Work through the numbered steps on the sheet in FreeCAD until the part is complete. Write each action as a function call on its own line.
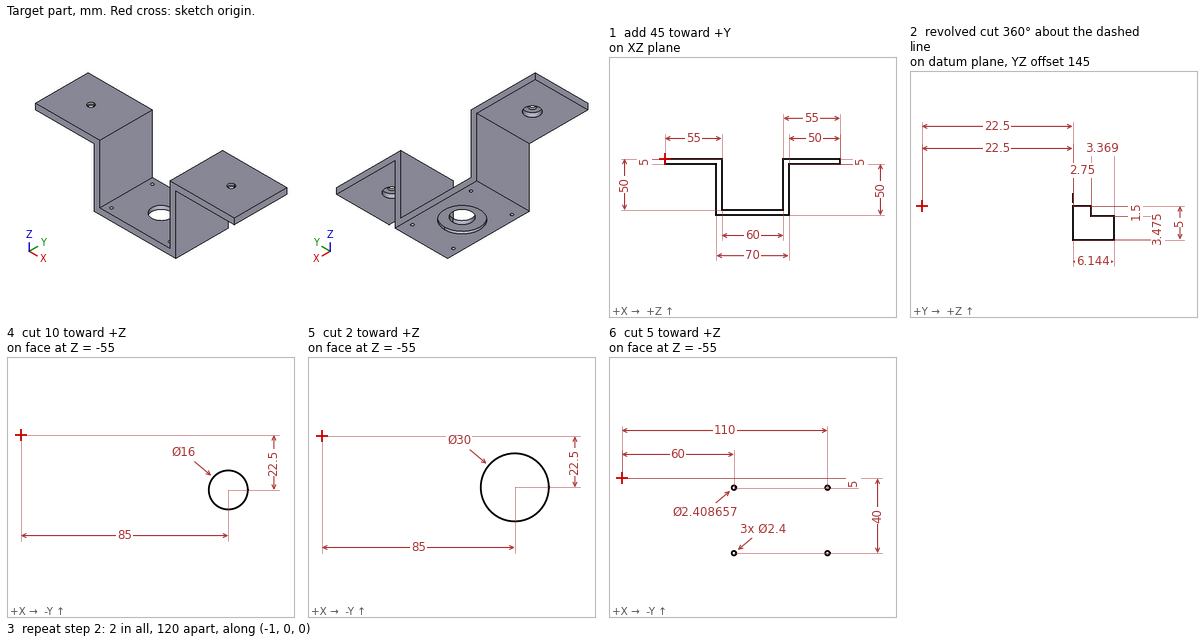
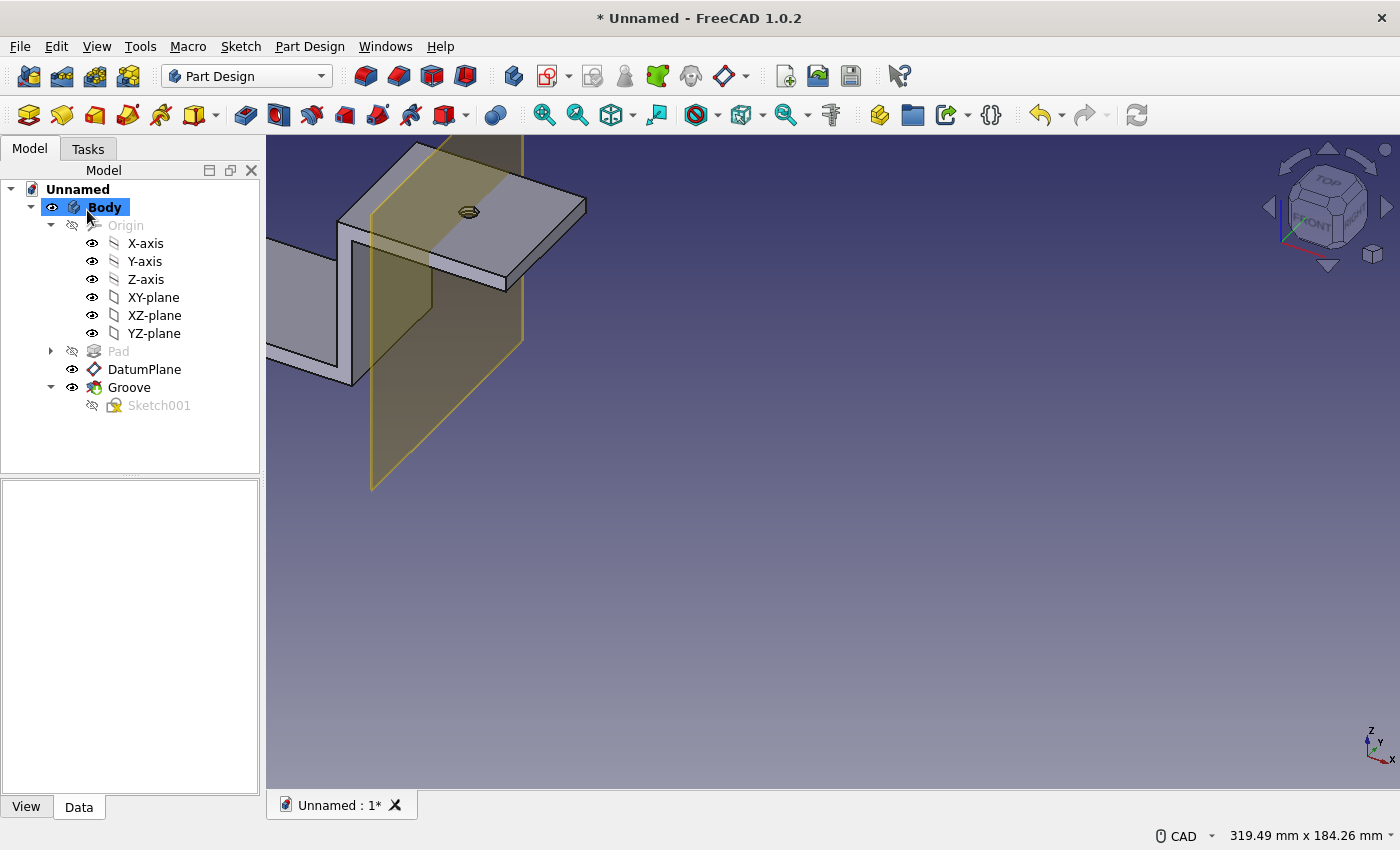
click(117, 369)
key(space)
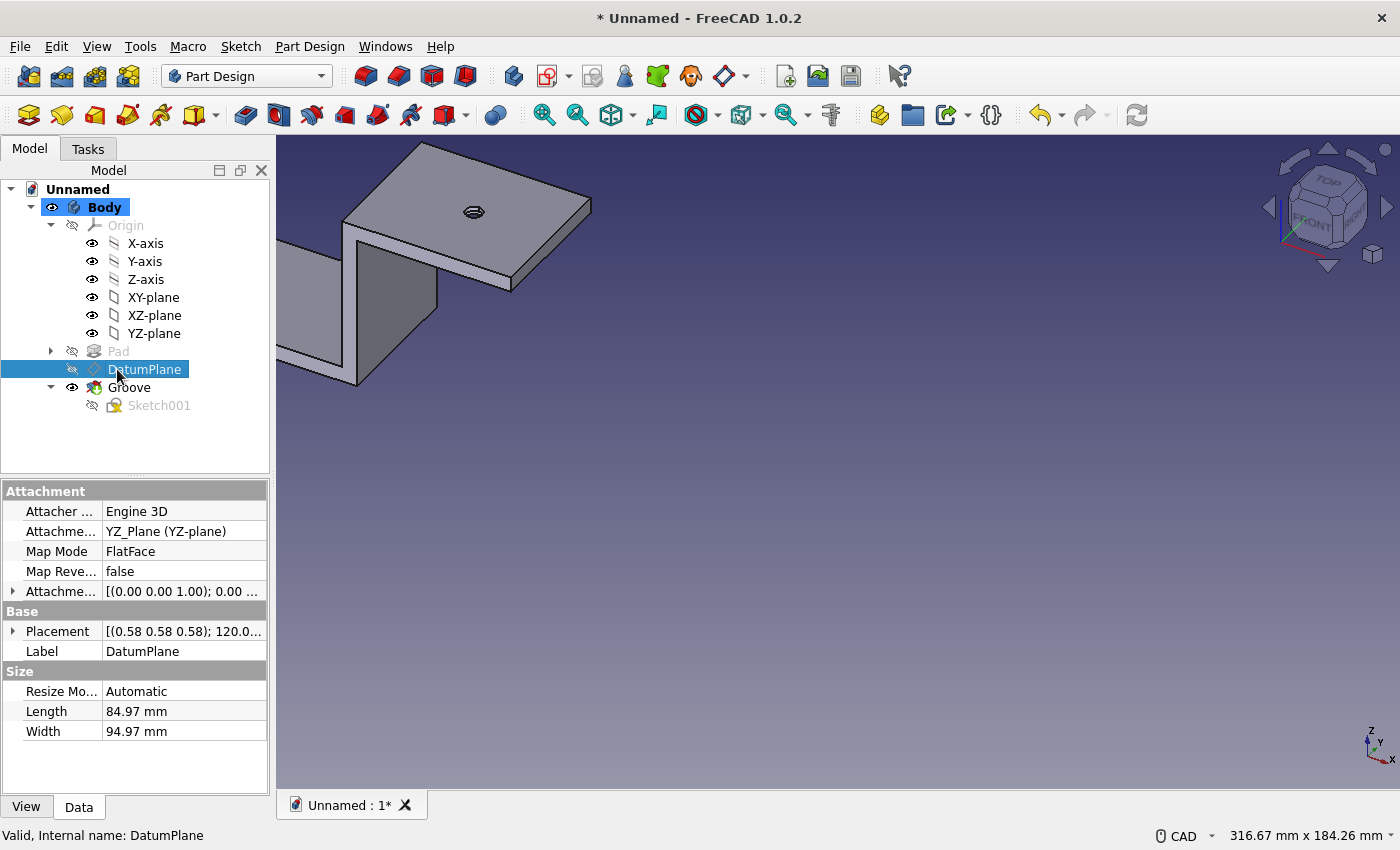
click(545, 116)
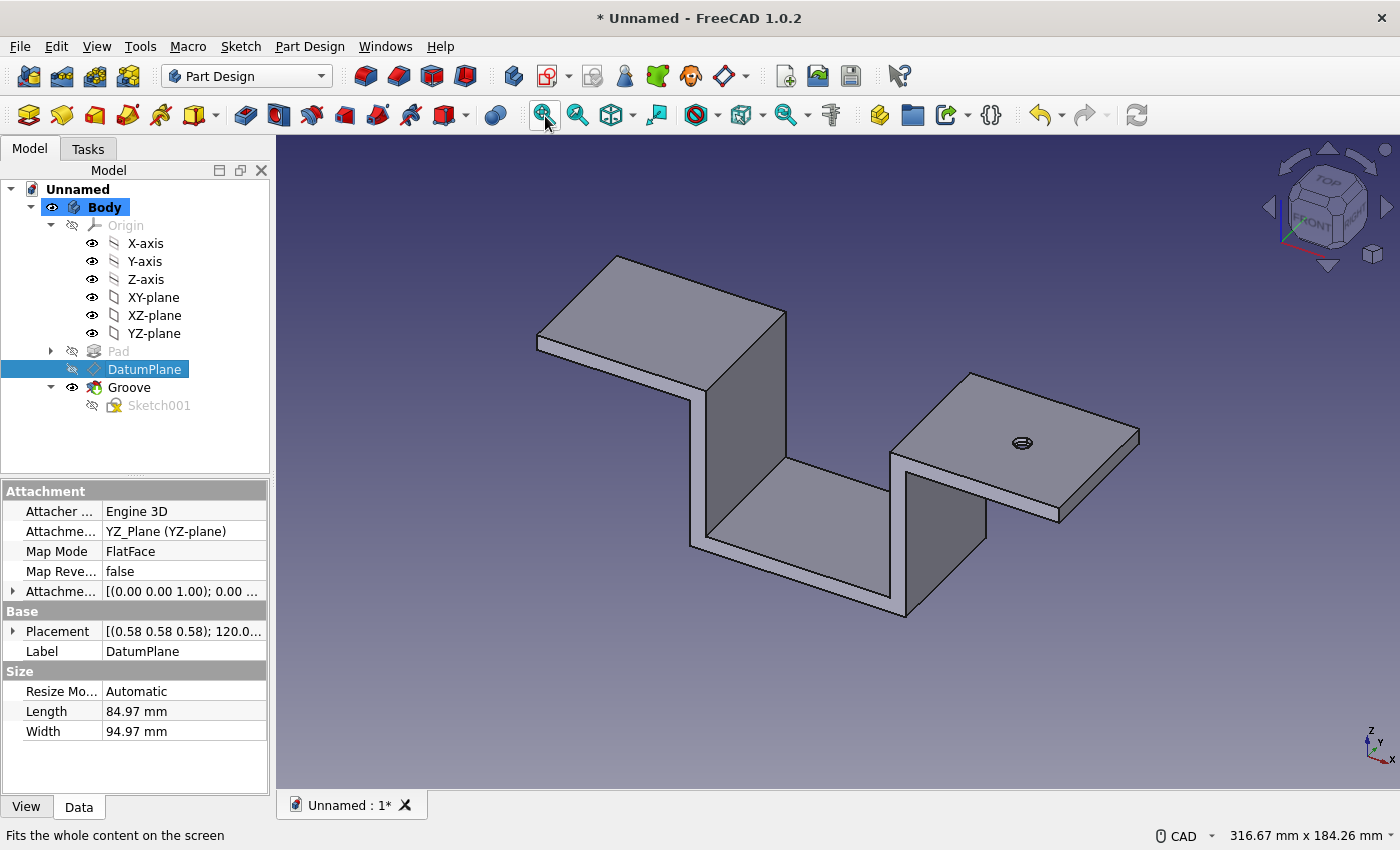
click(117, 387)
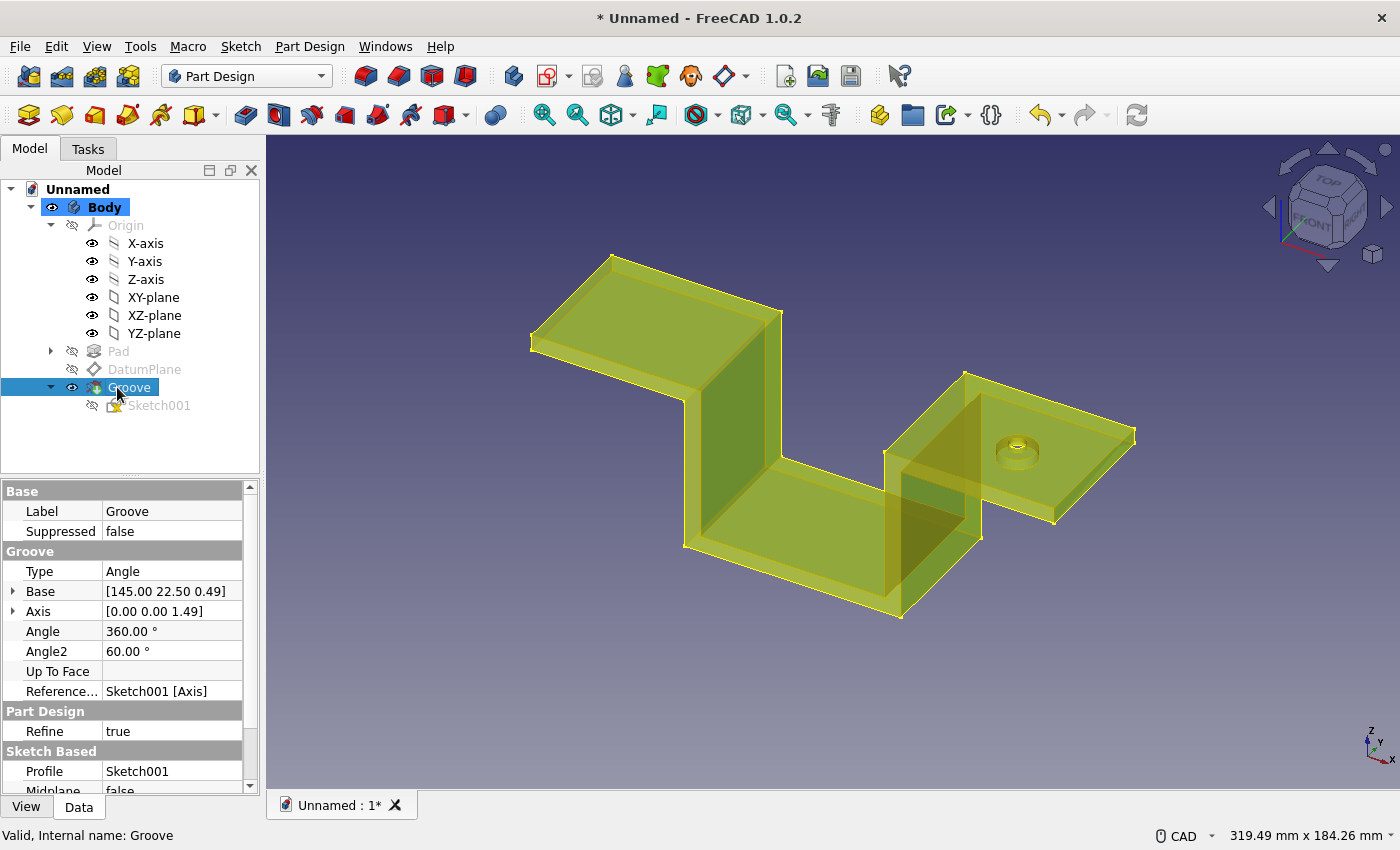
click(62, 76)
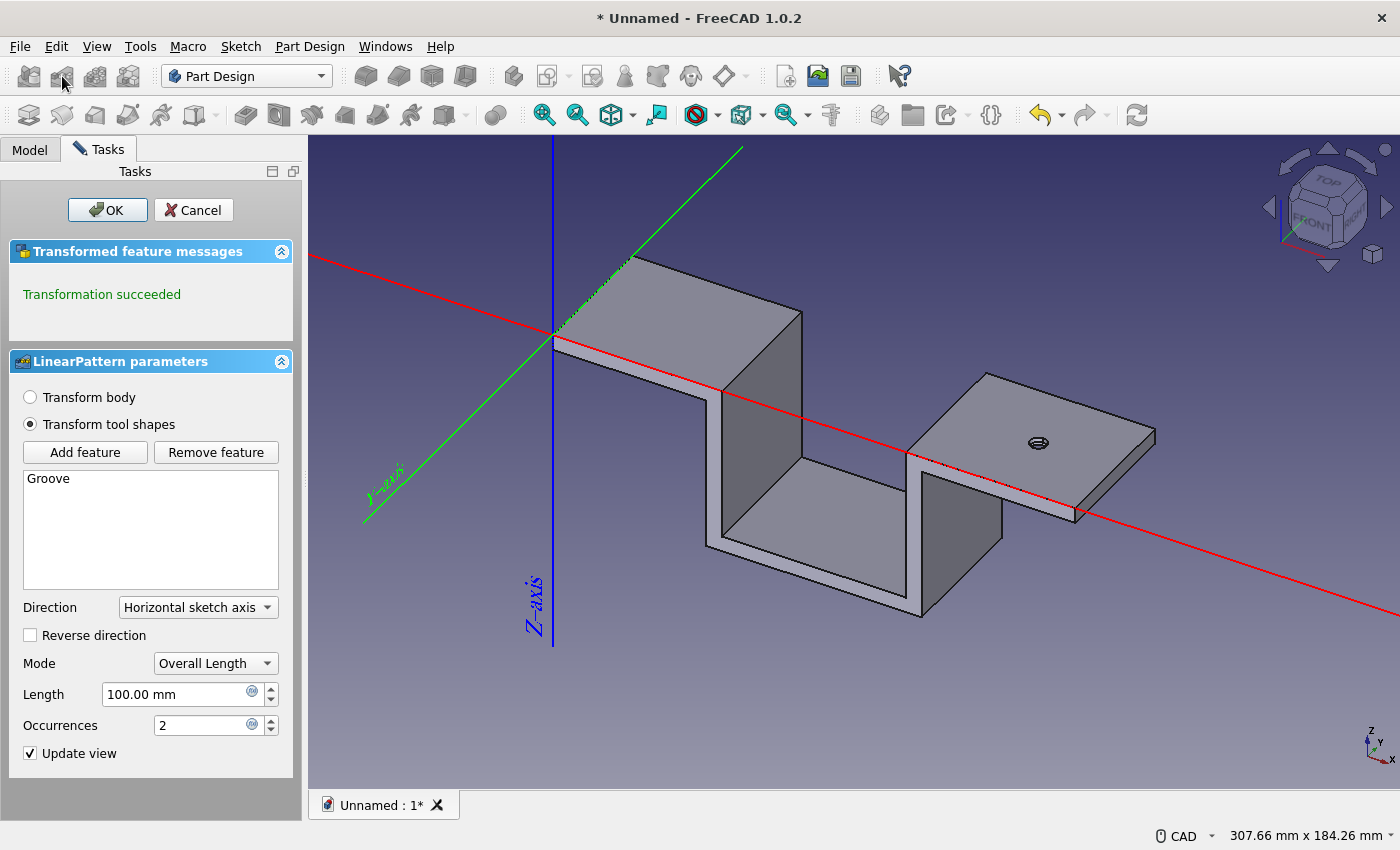
click(199, 608)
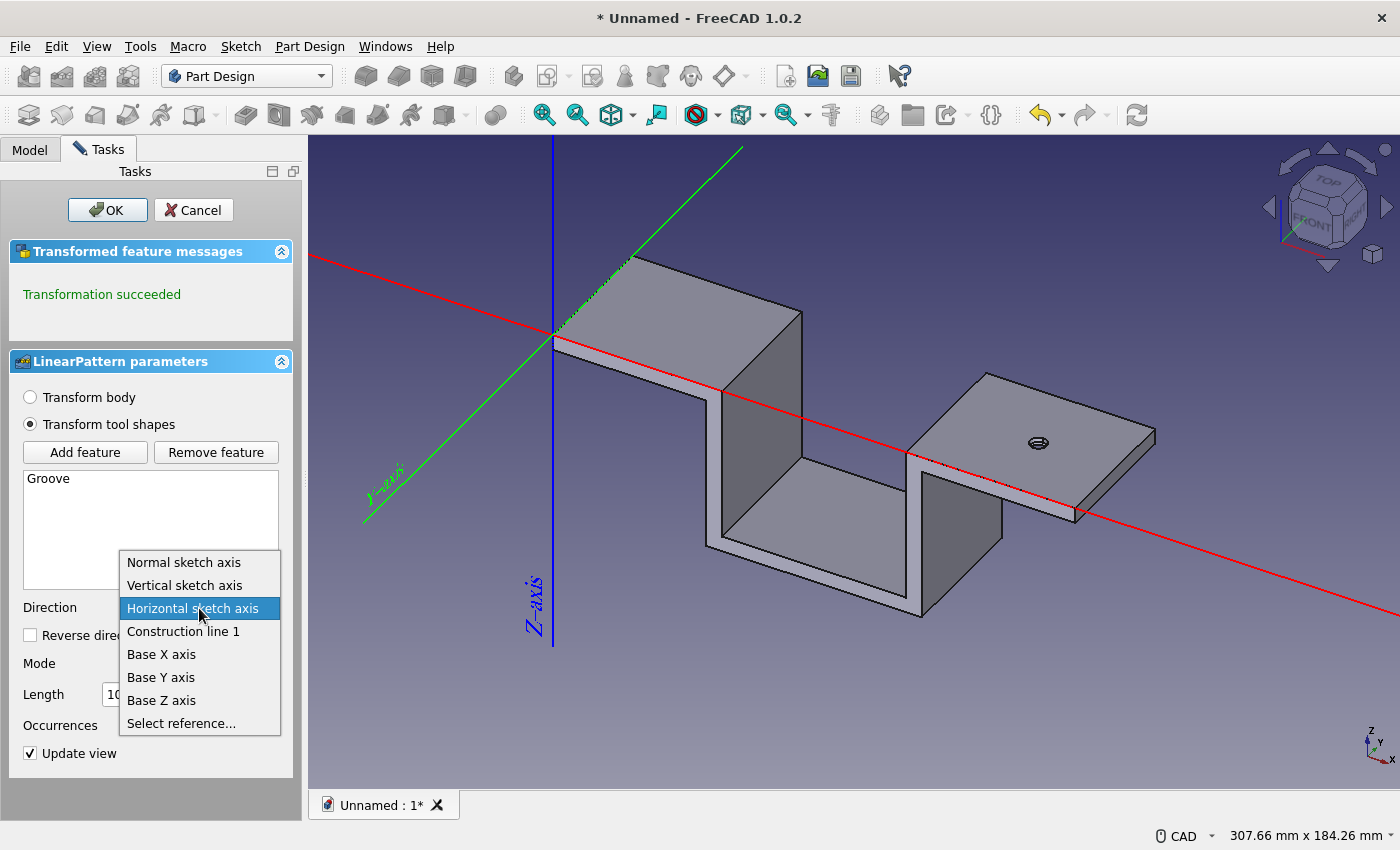
click(198, 654)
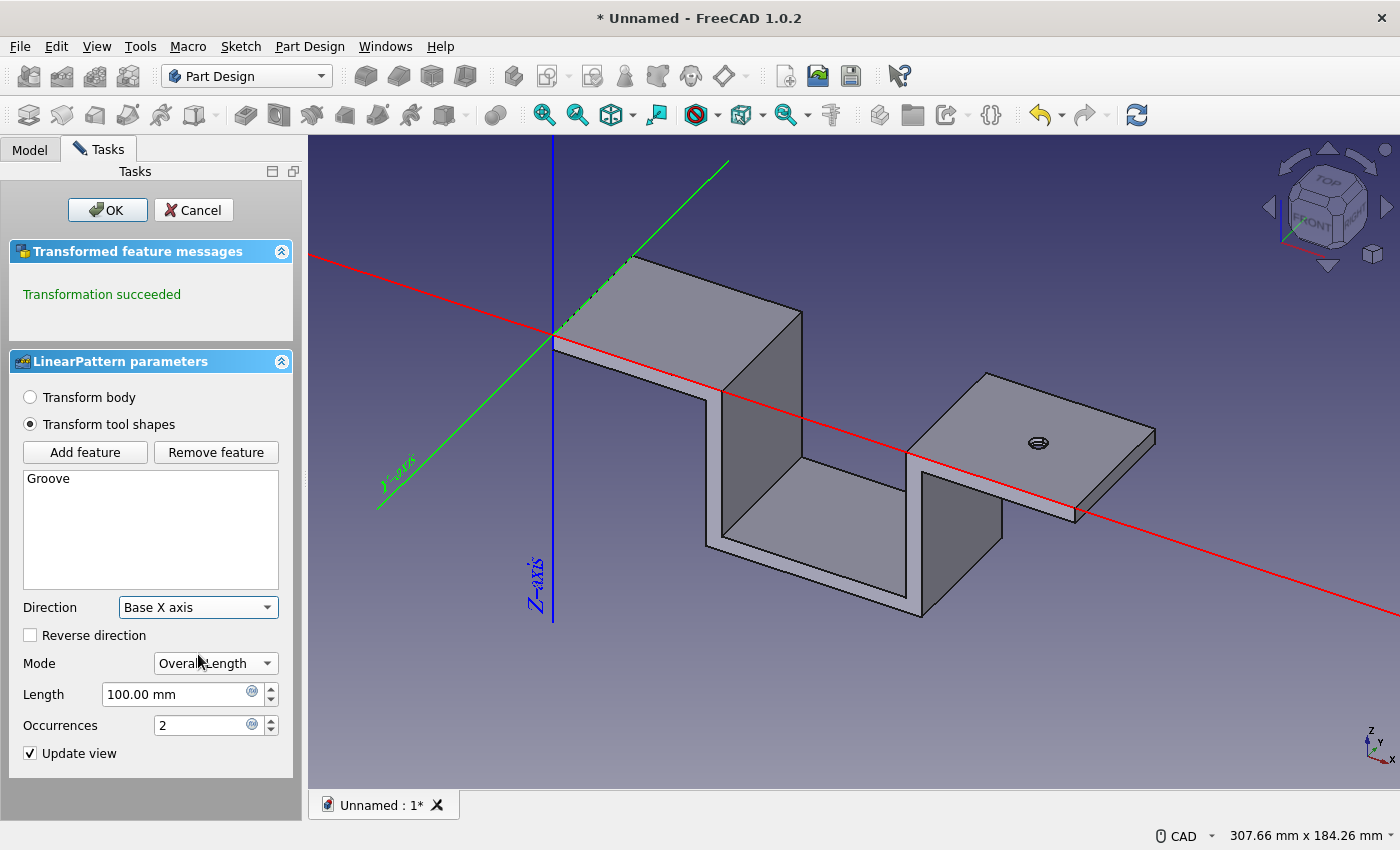
click(216, 664)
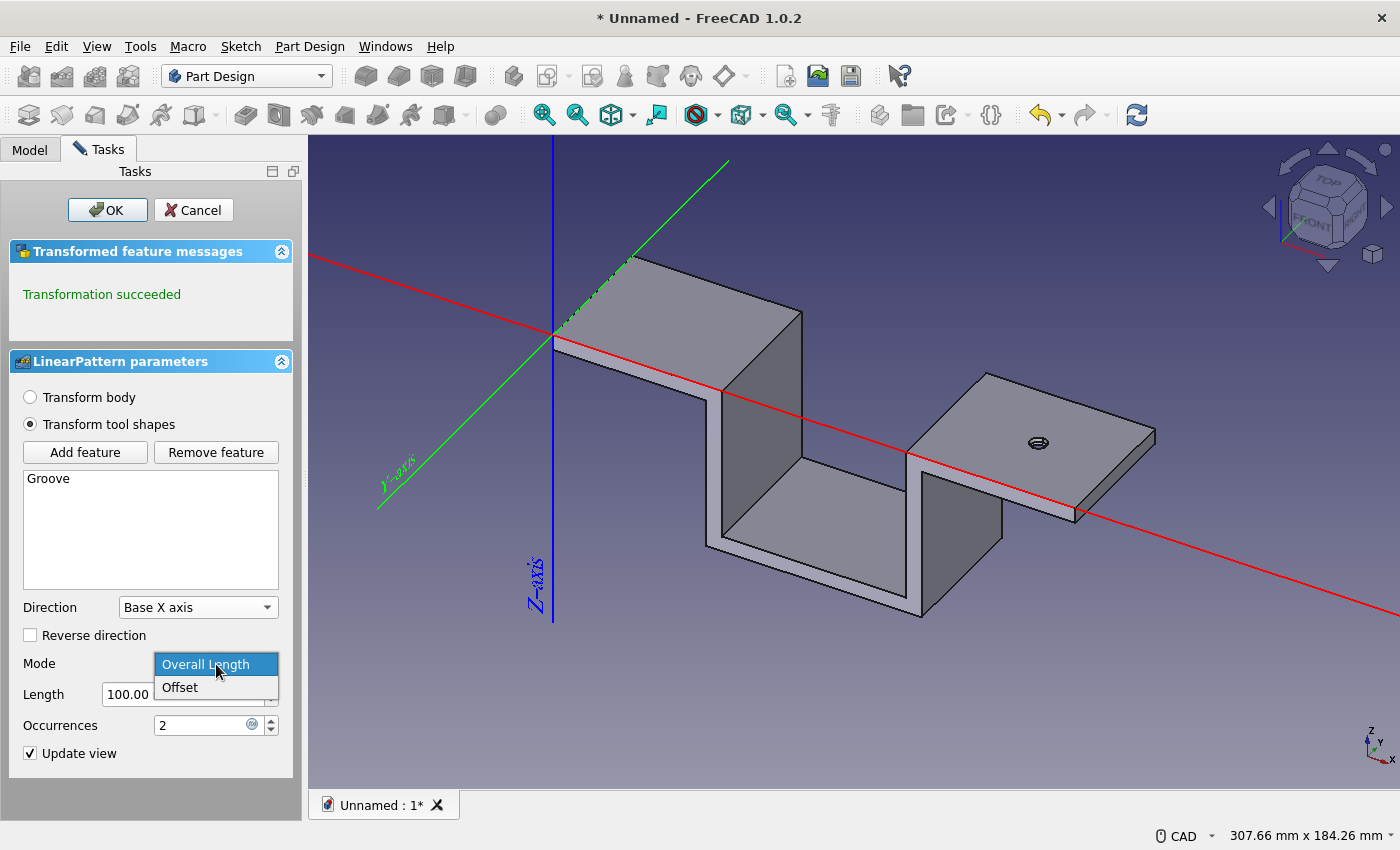
click(214, 688)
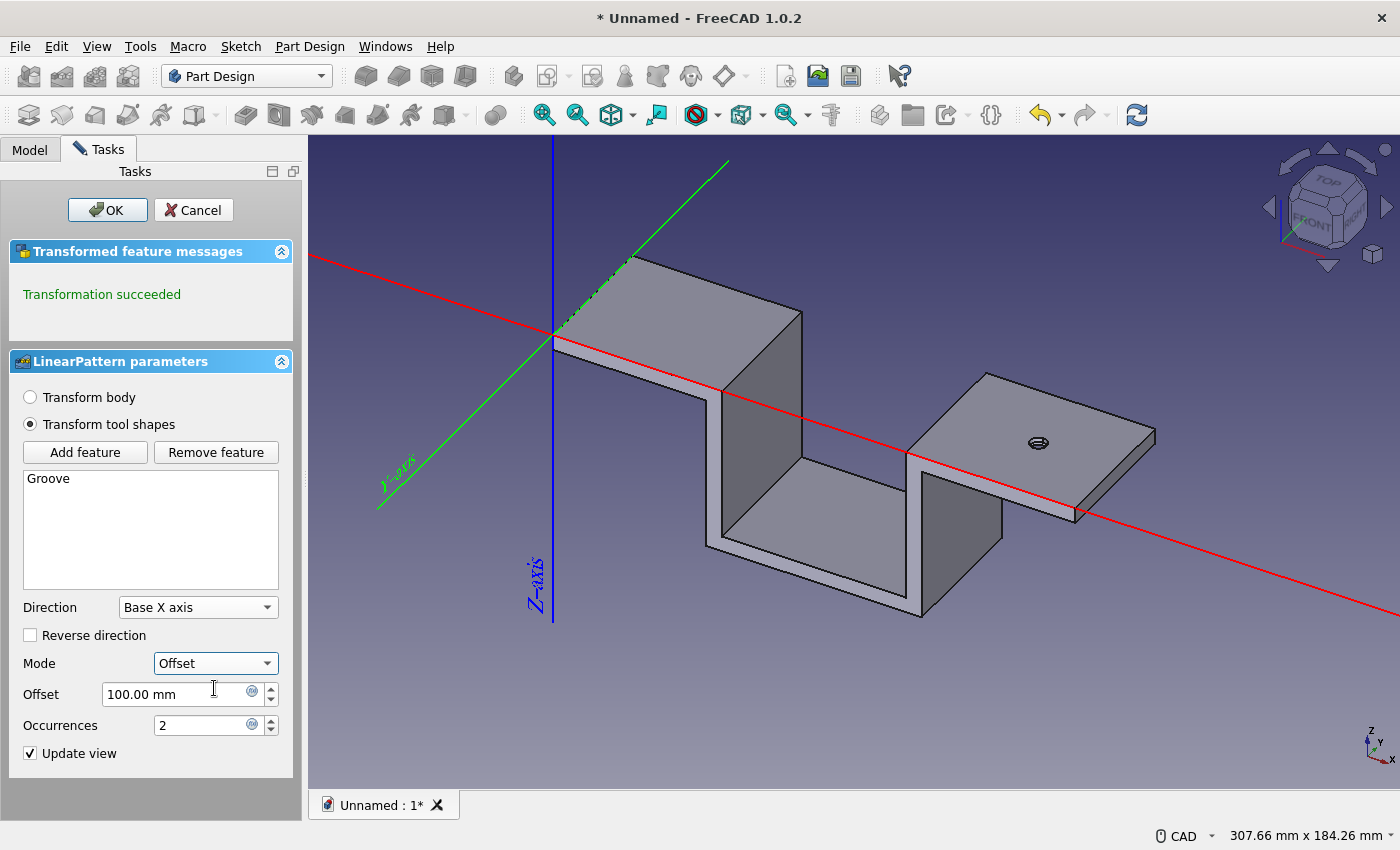
triple_click(184, 694)